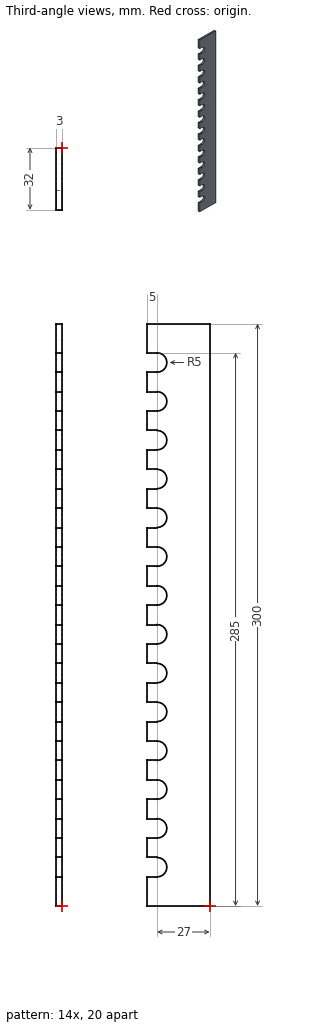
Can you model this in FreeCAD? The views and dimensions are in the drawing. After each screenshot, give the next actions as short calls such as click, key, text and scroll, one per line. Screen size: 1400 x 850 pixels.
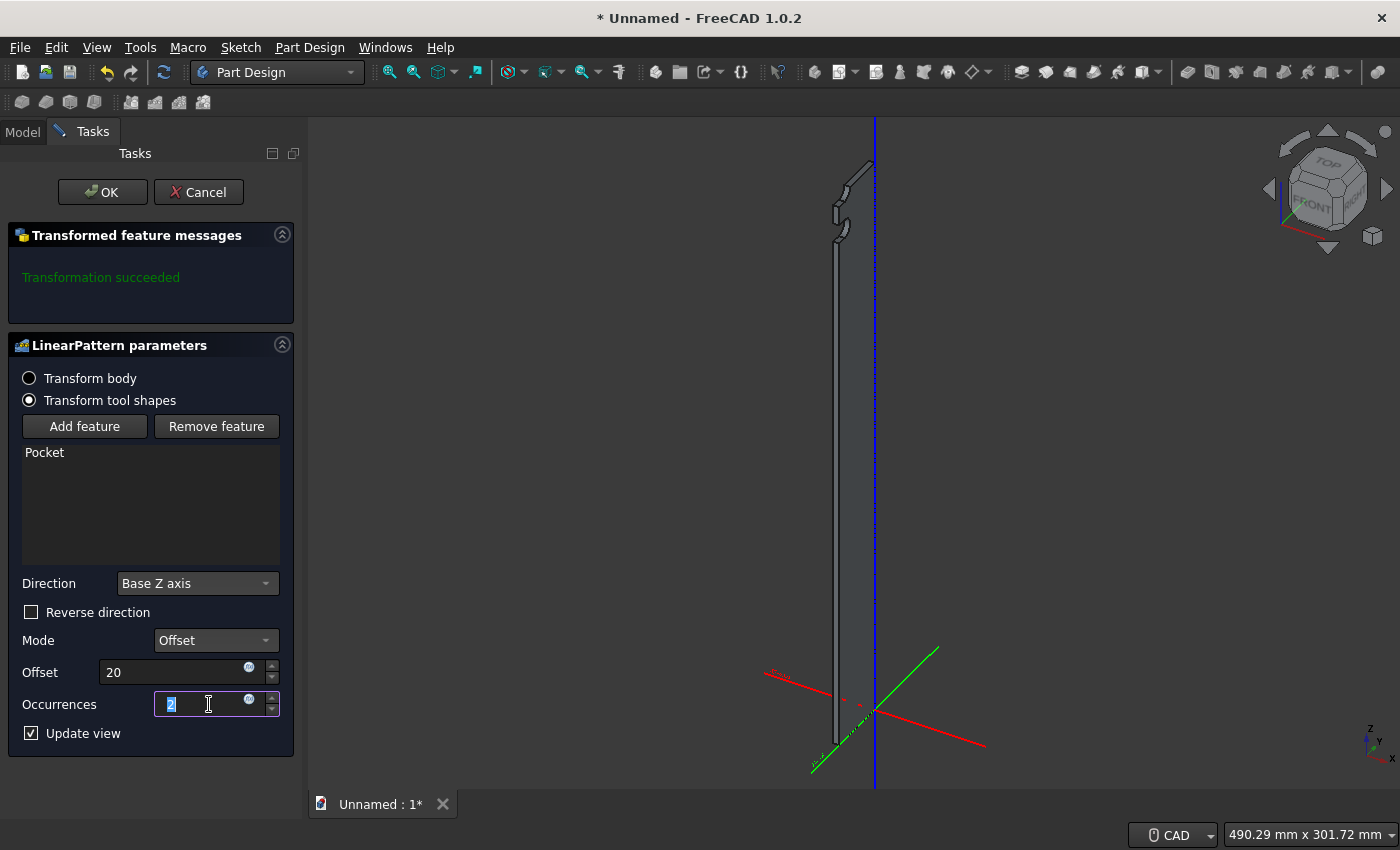
text(14)
key(Tab)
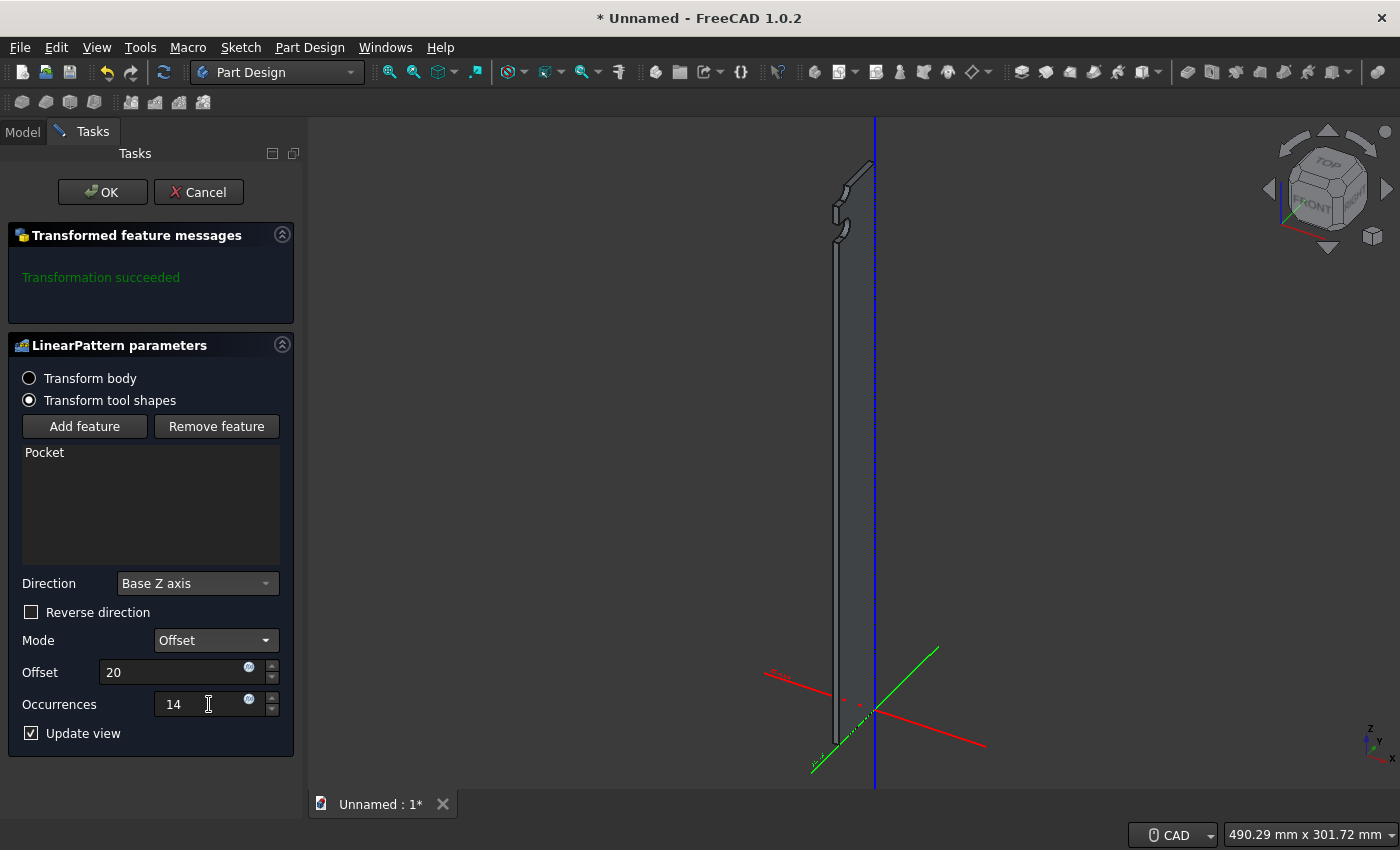
click(30, 612)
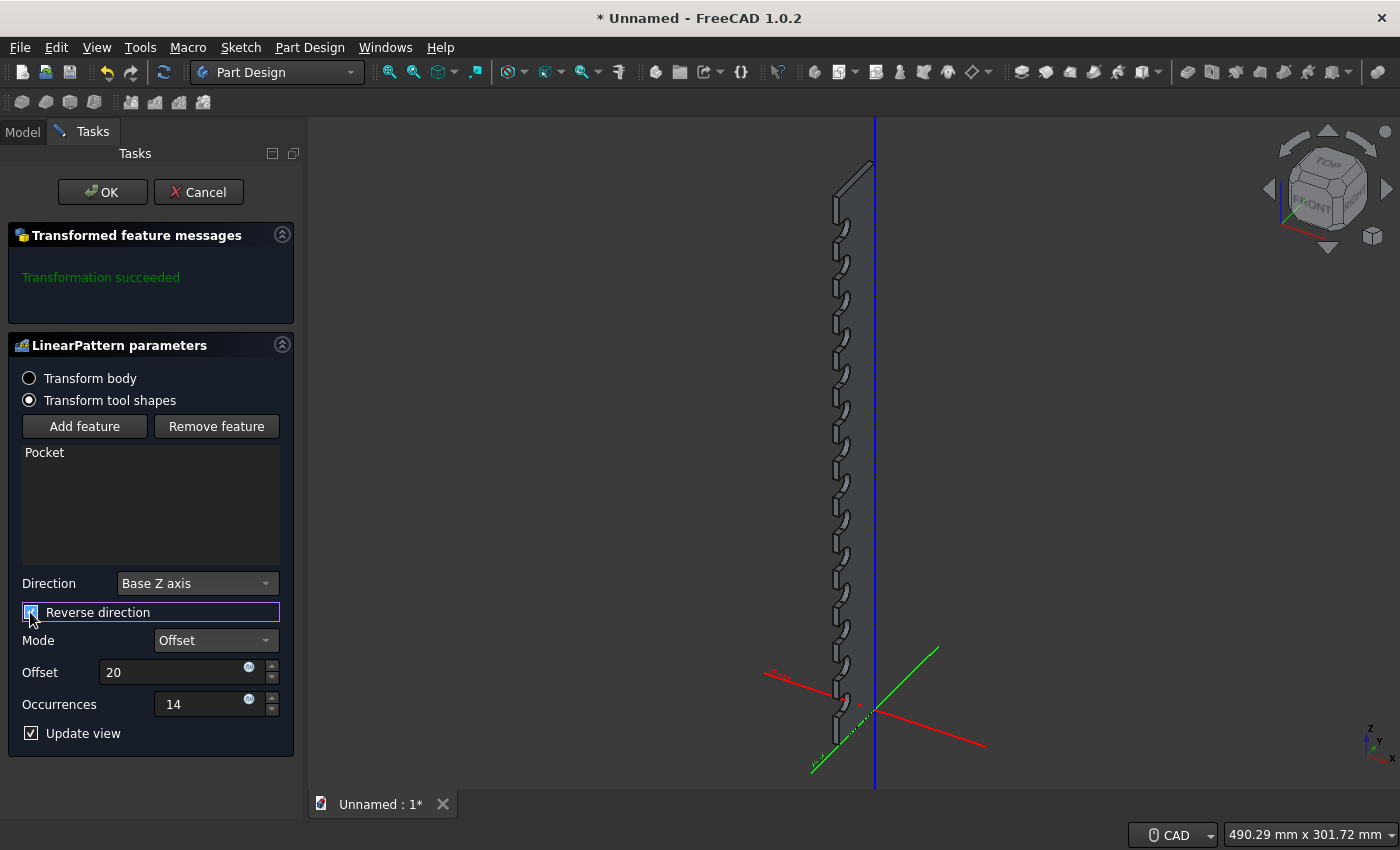
click(103, 192)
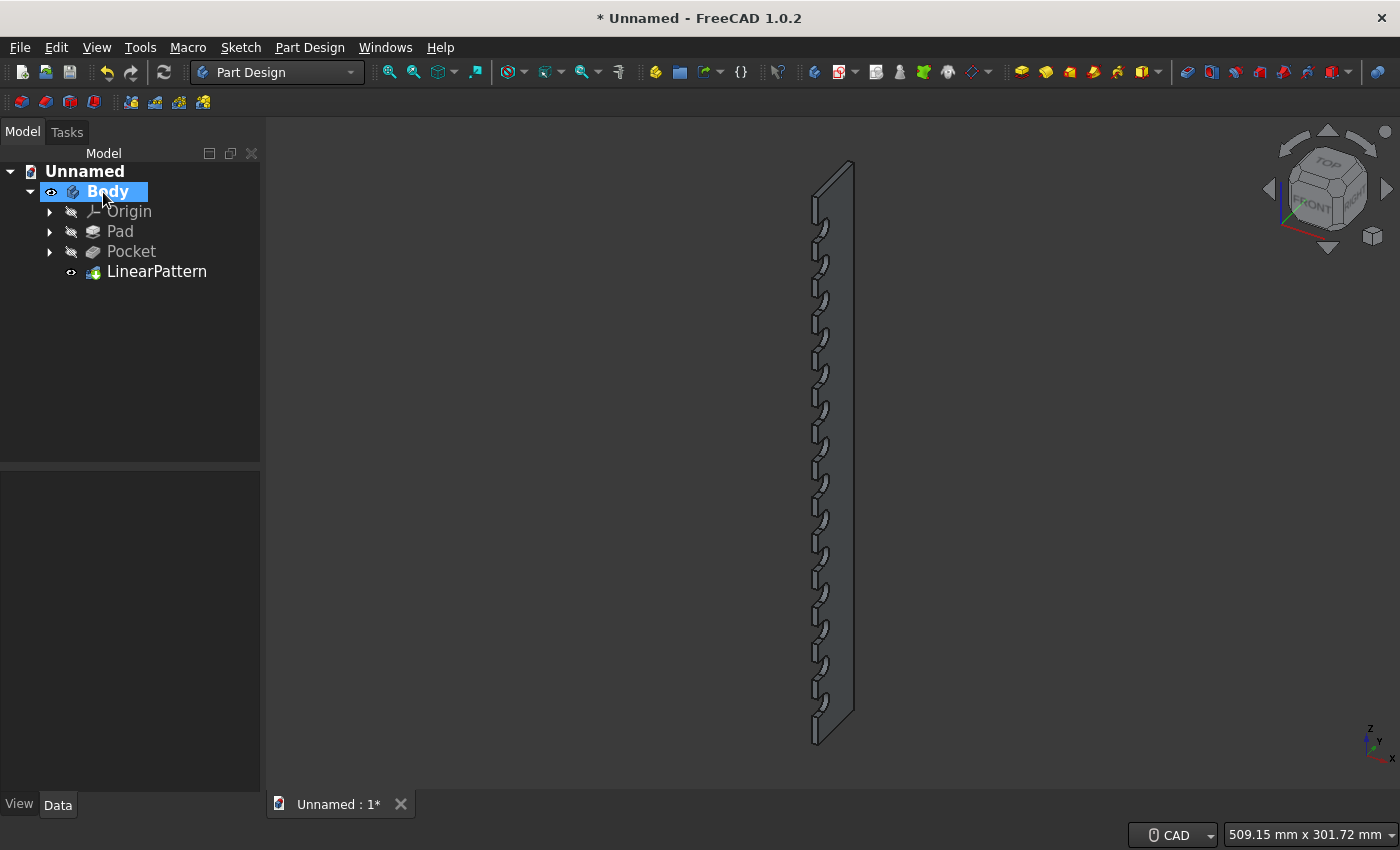
key(0)